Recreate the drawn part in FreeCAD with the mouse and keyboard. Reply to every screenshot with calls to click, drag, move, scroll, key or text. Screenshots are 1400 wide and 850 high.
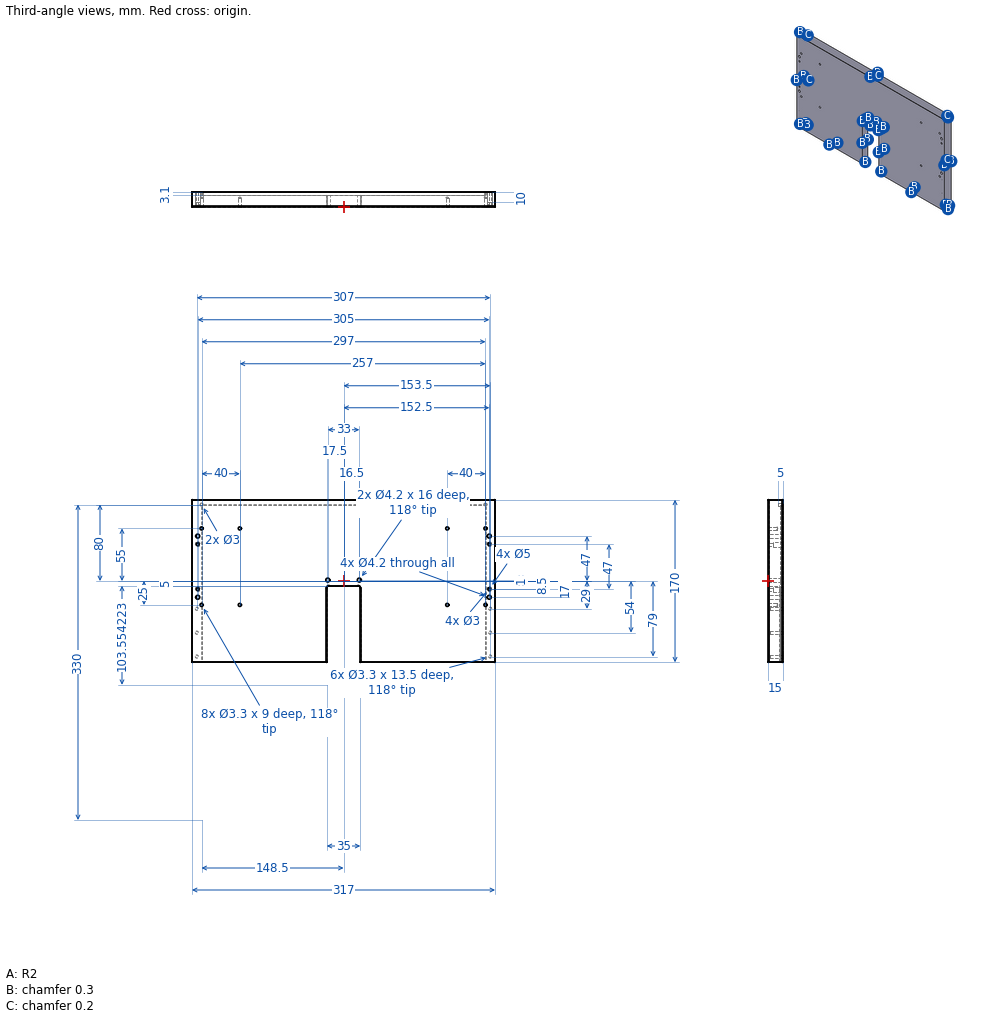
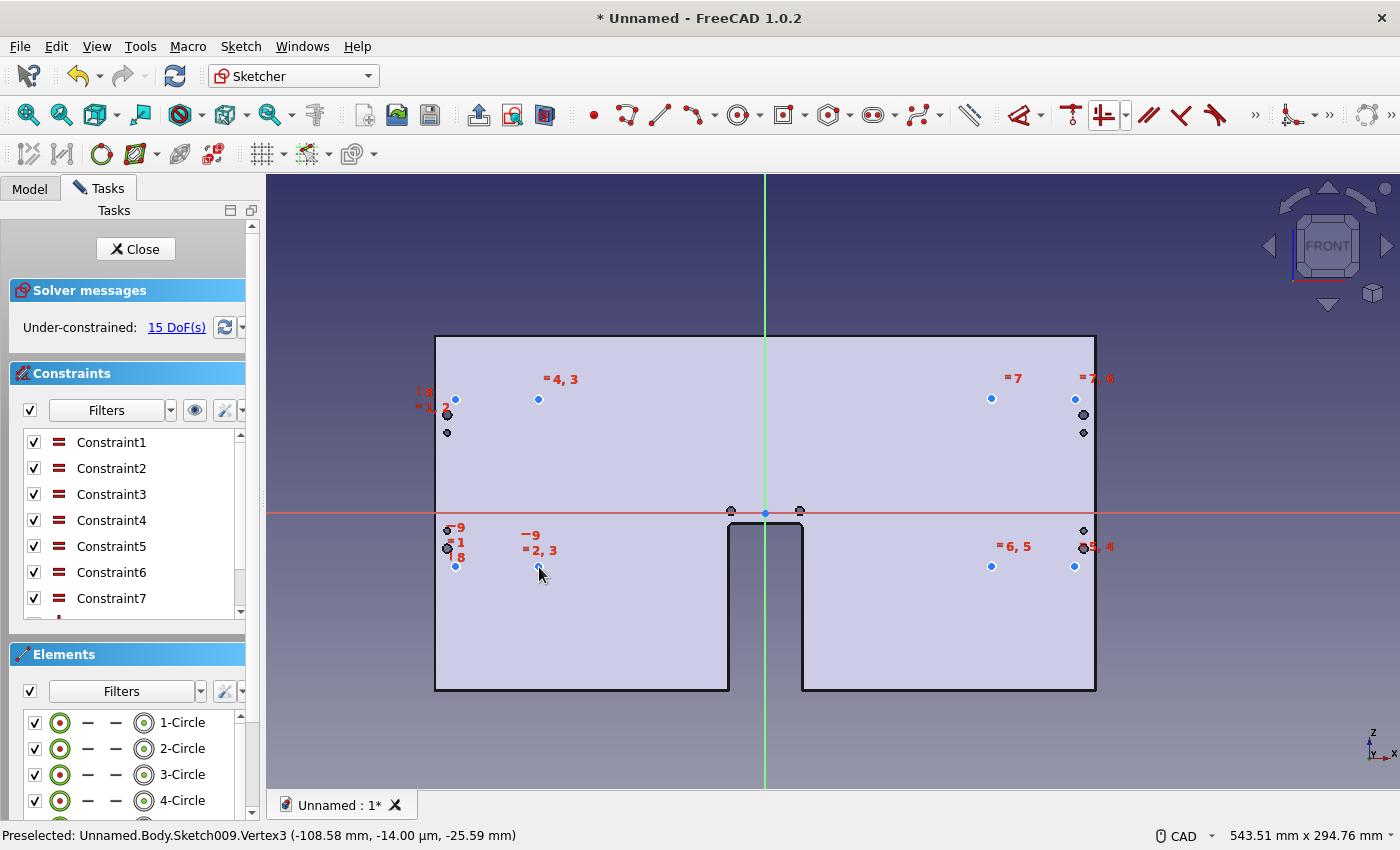
click(539, 567)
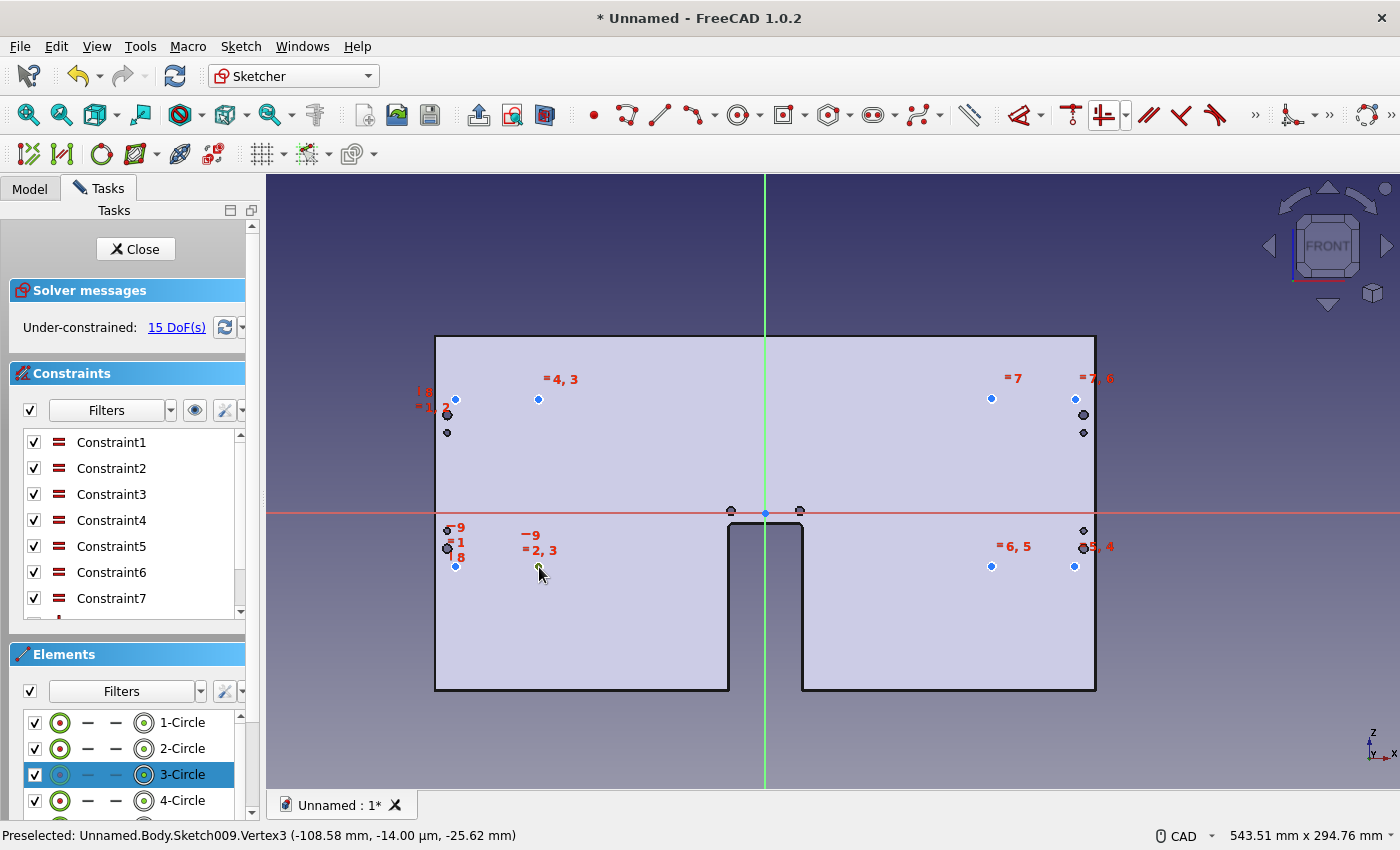
click(539, 399)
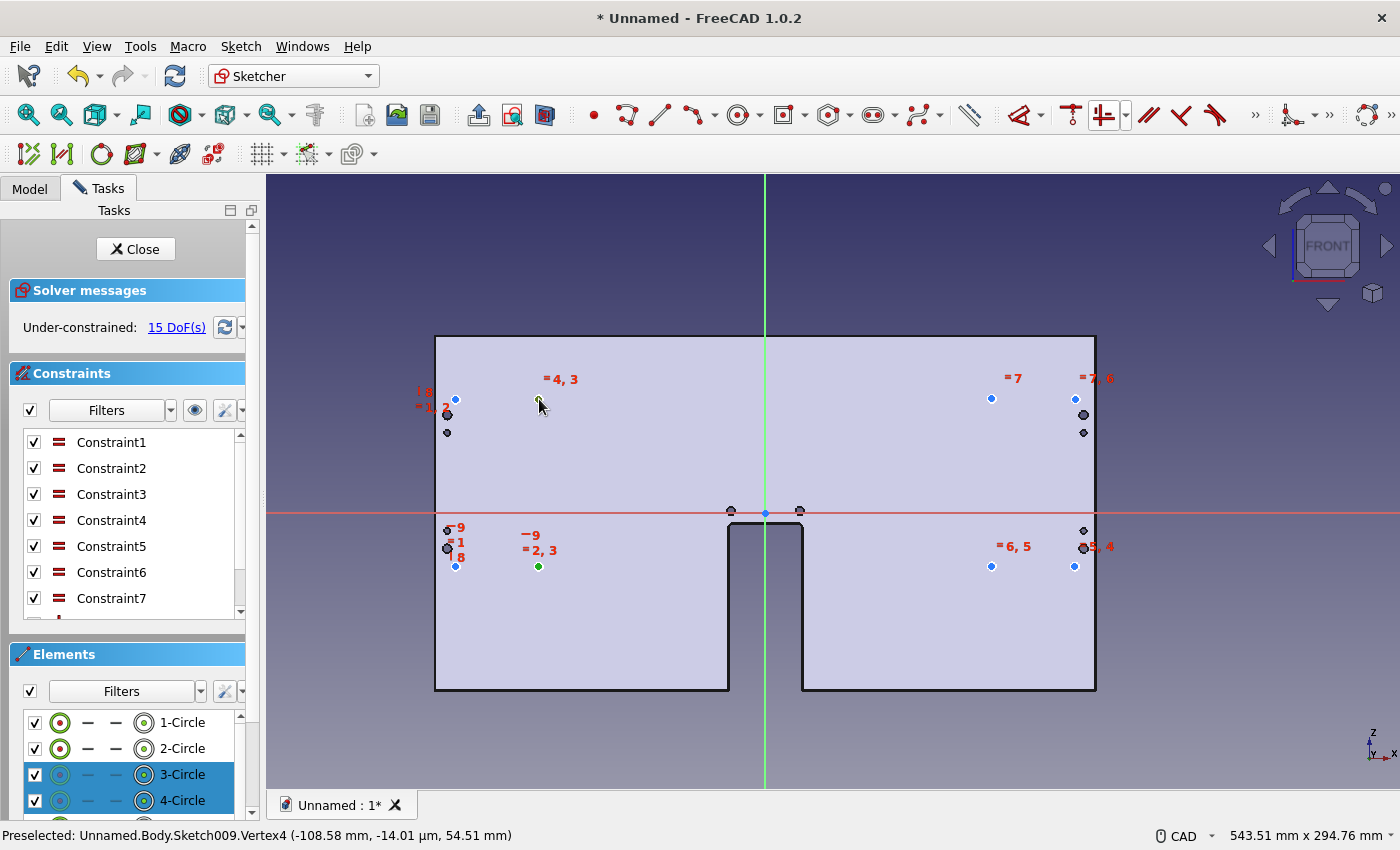
key(v)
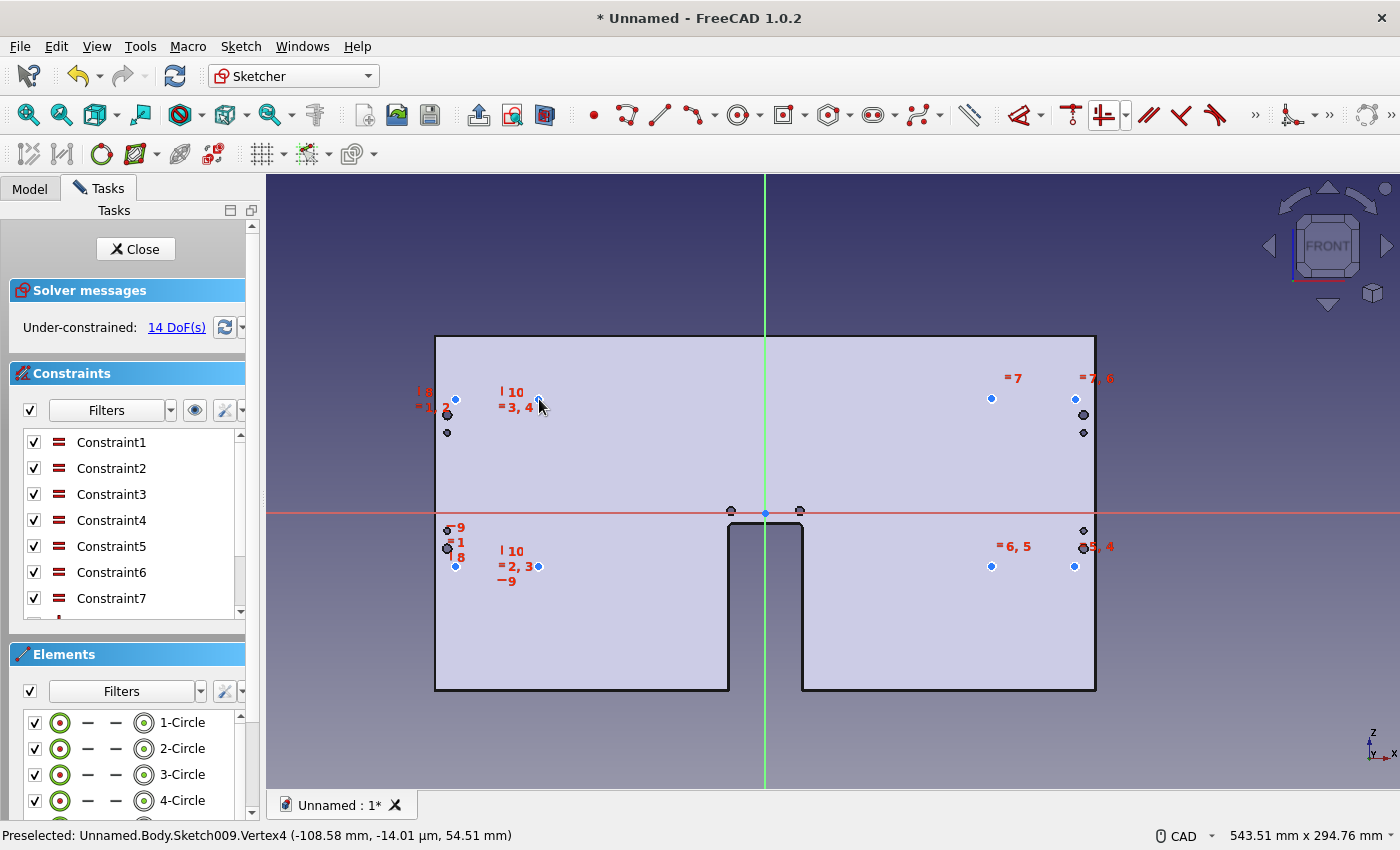
click(456, 400)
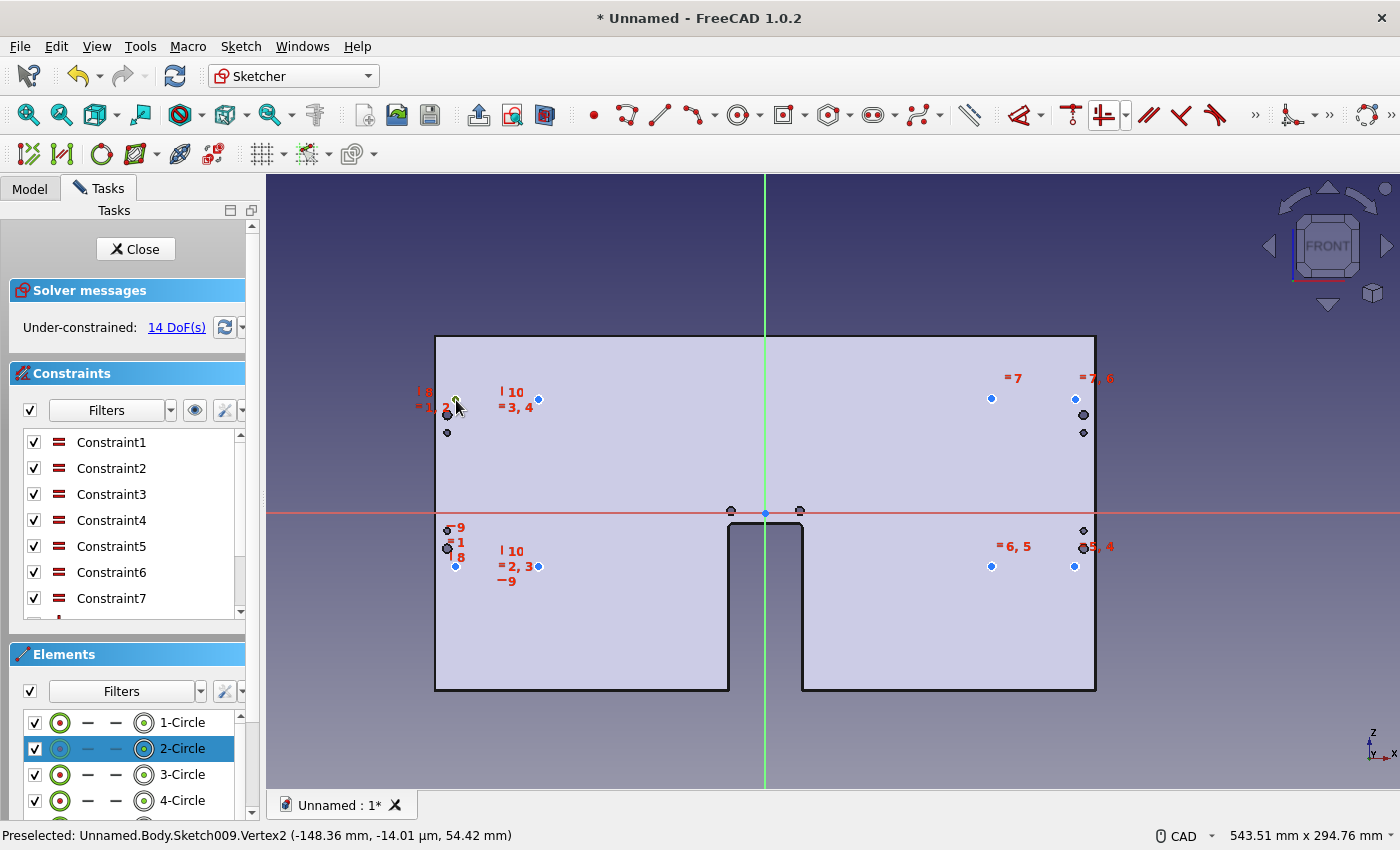
click(539, 399)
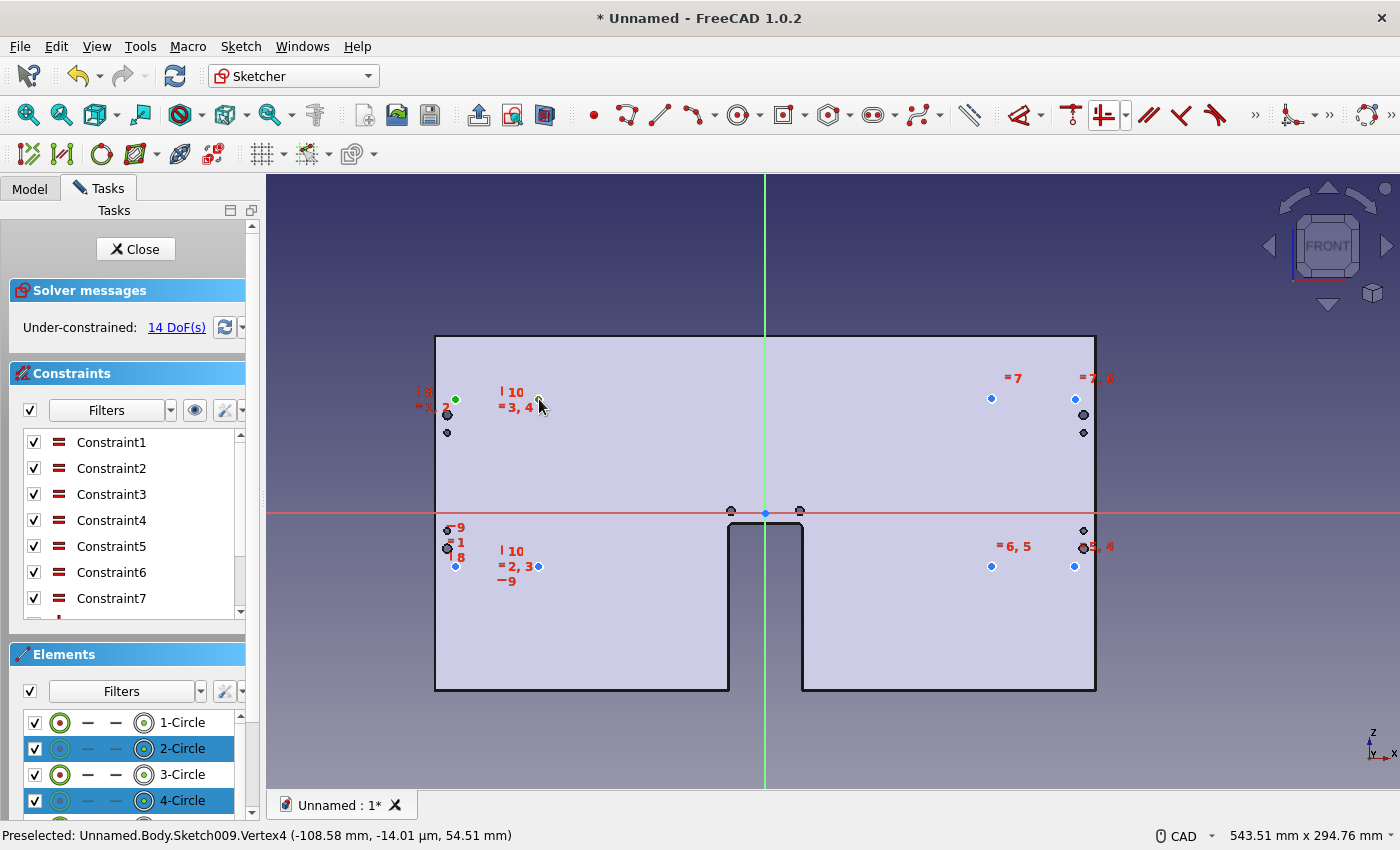
key(h)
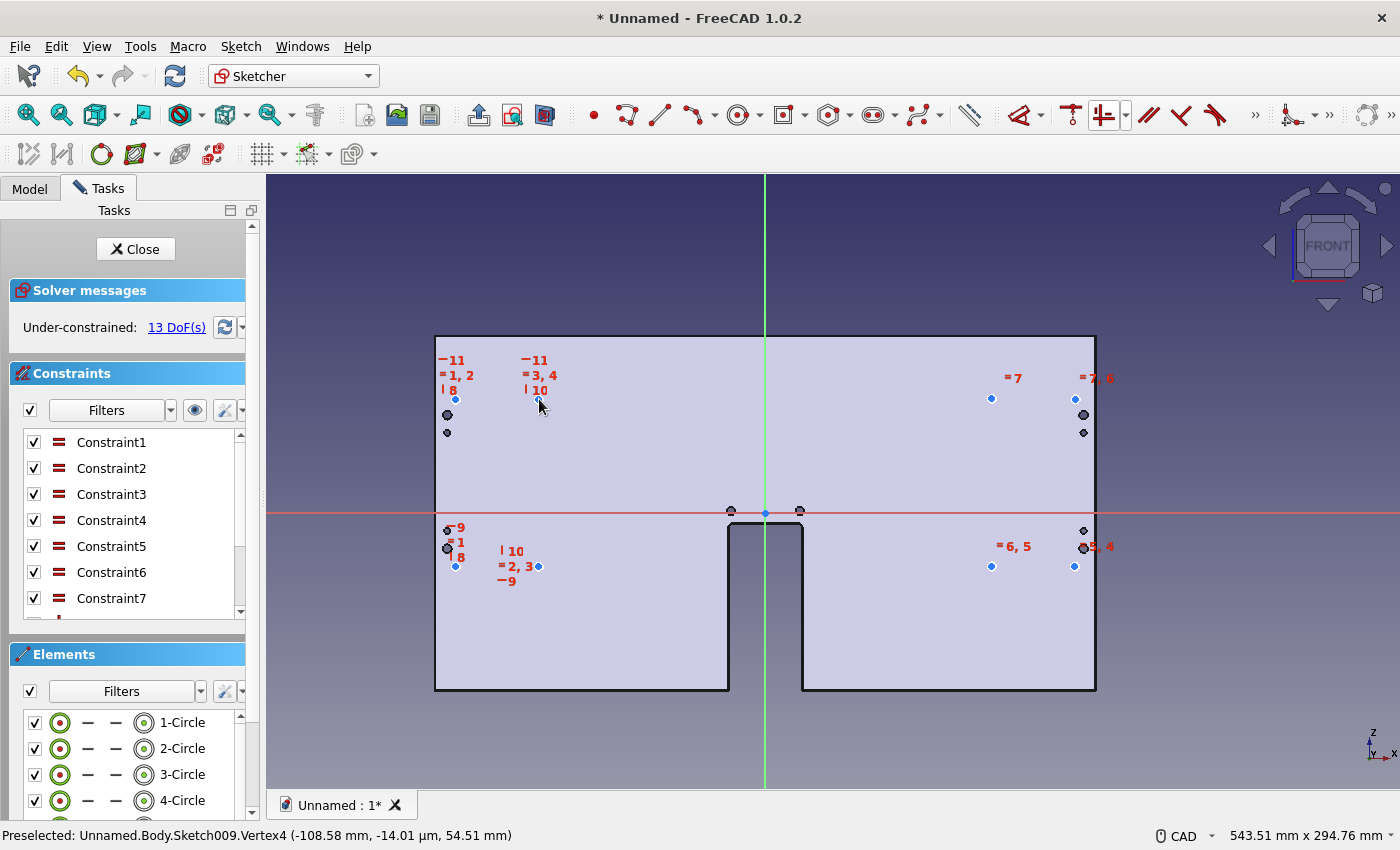
click(539, 567)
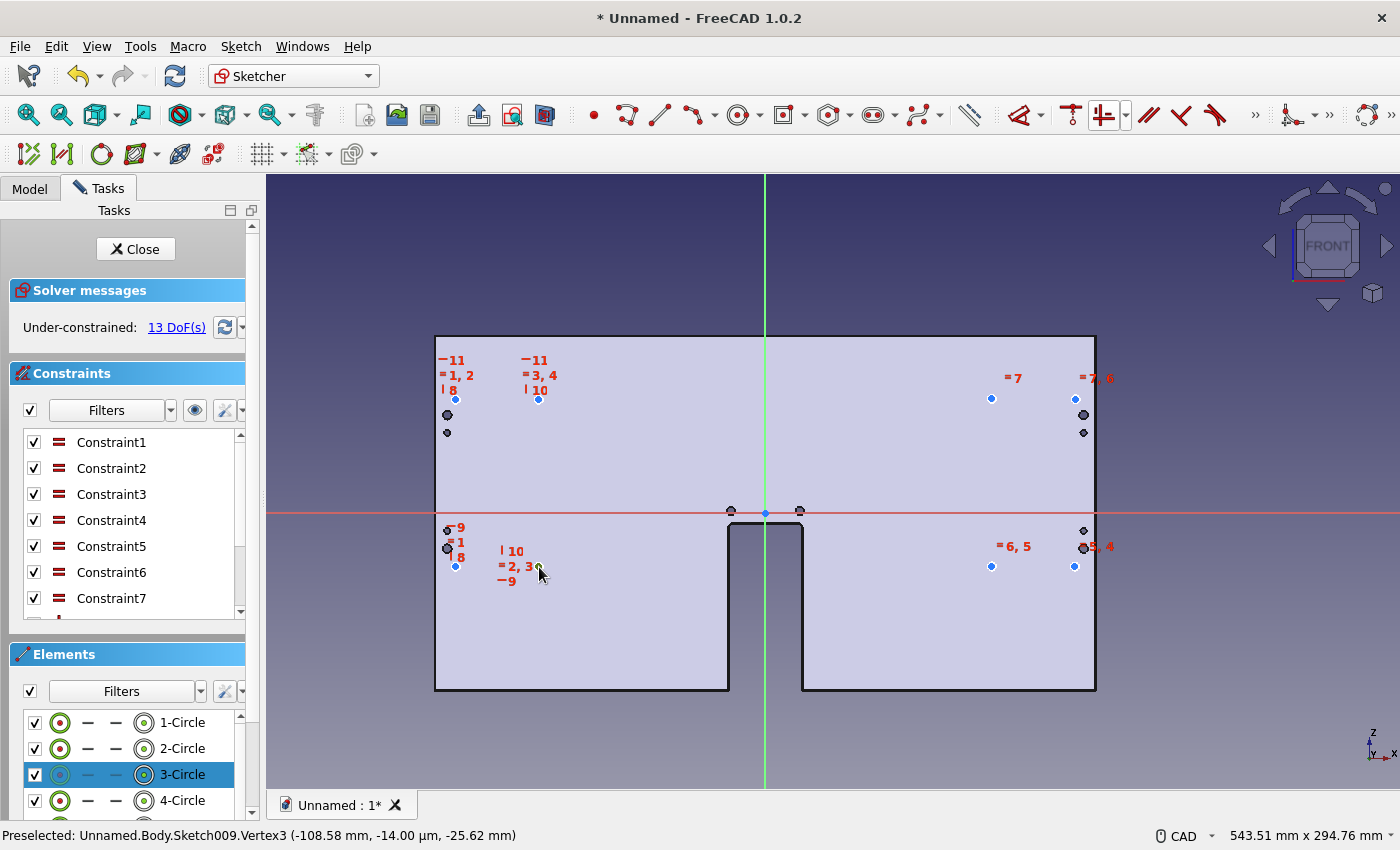
click(1075, 567)